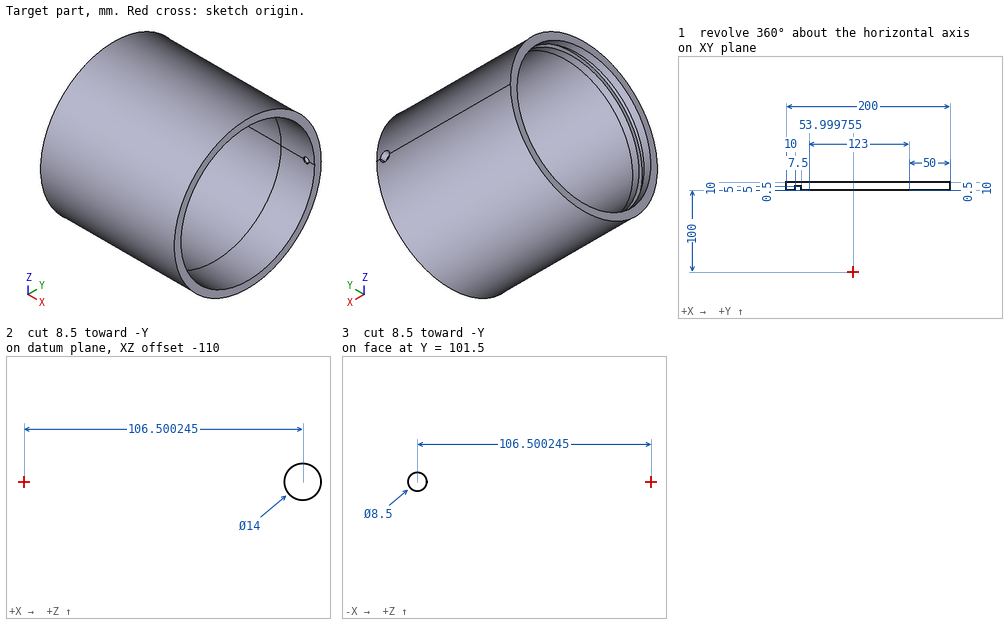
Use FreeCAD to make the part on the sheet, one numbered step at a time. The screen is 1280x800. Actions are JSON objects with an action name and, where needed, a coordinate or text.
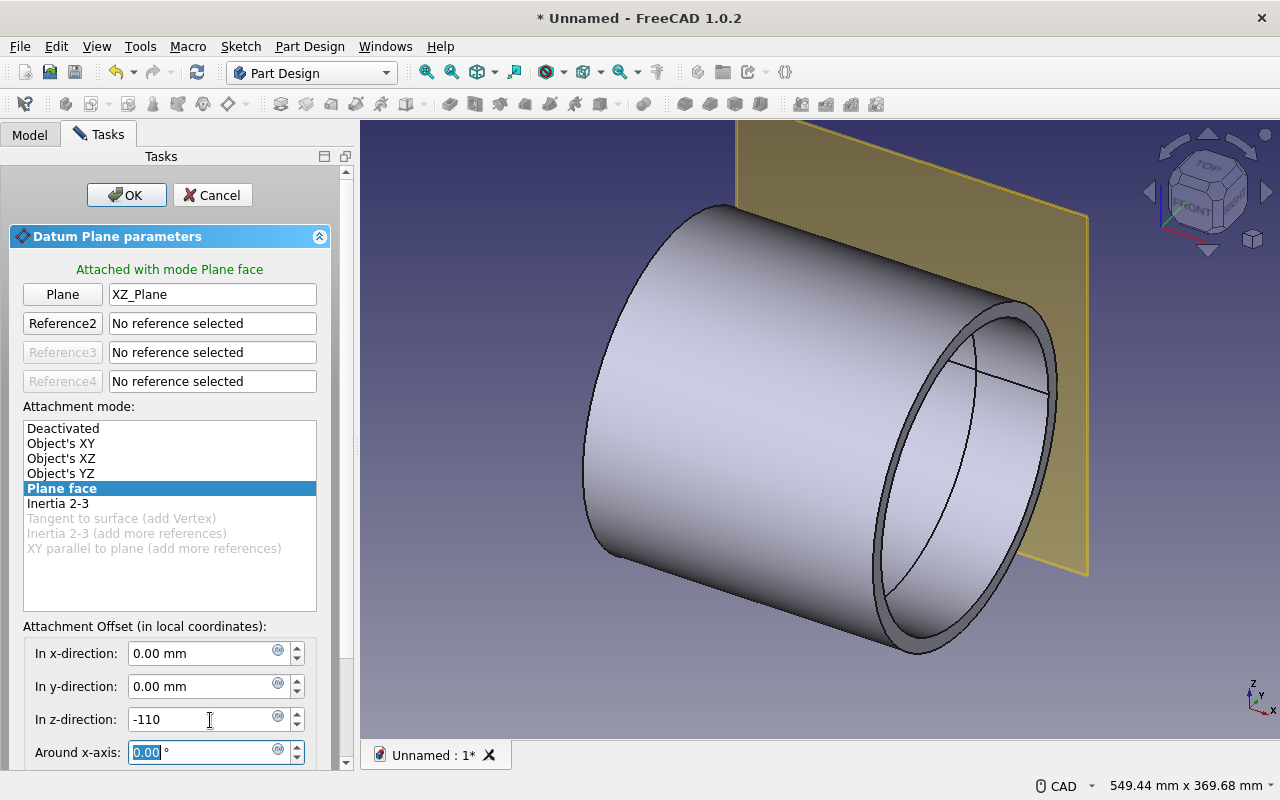
{"action": "left_click", "coordinate": [127, 195]}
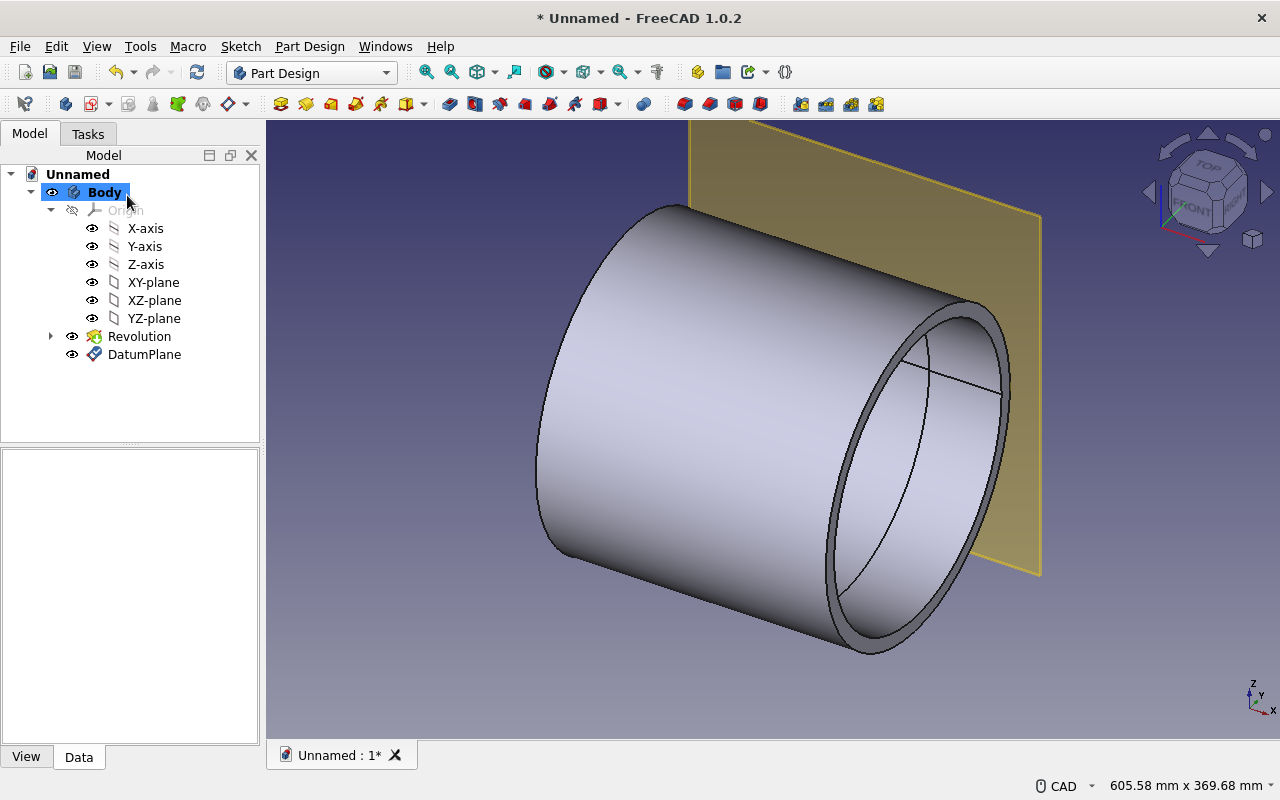
{"action": "left_click", "coordinate": [117, 354]}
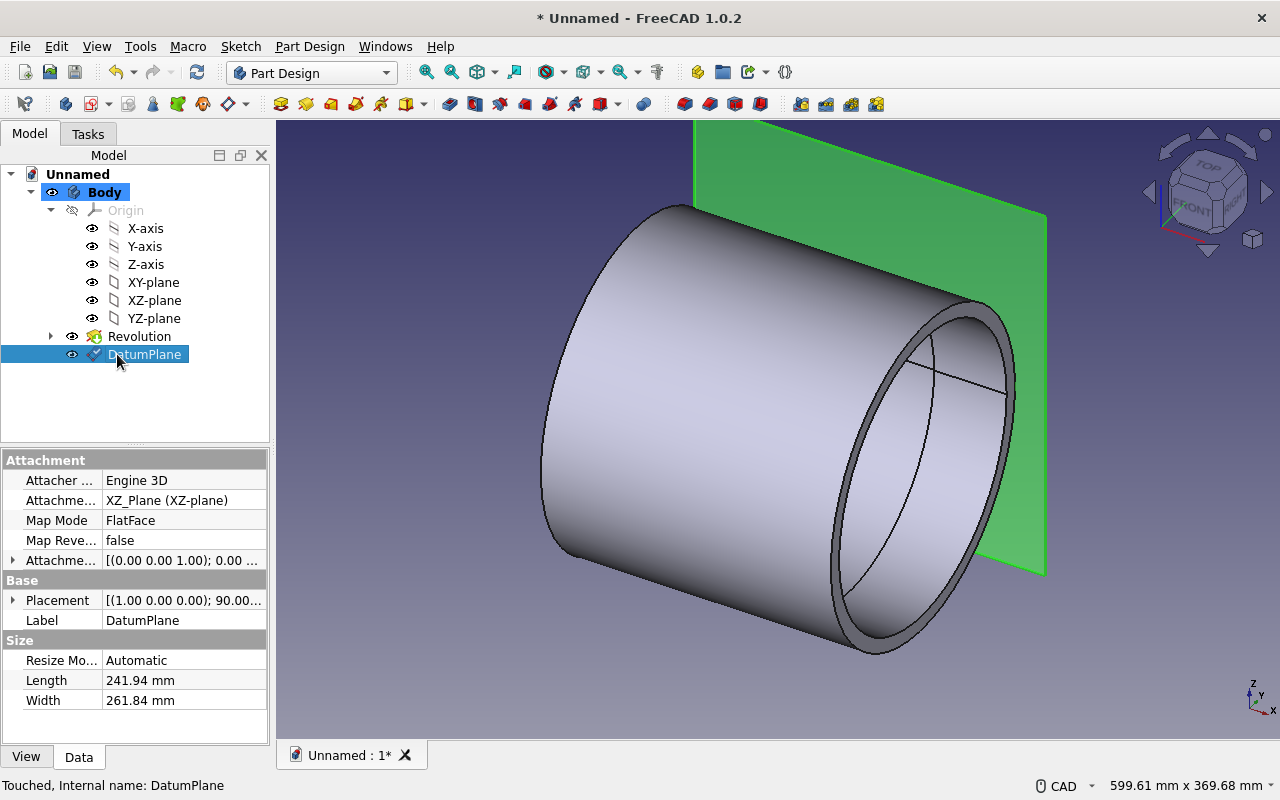
{"action": "left_click", "coordinate": [90, 104]}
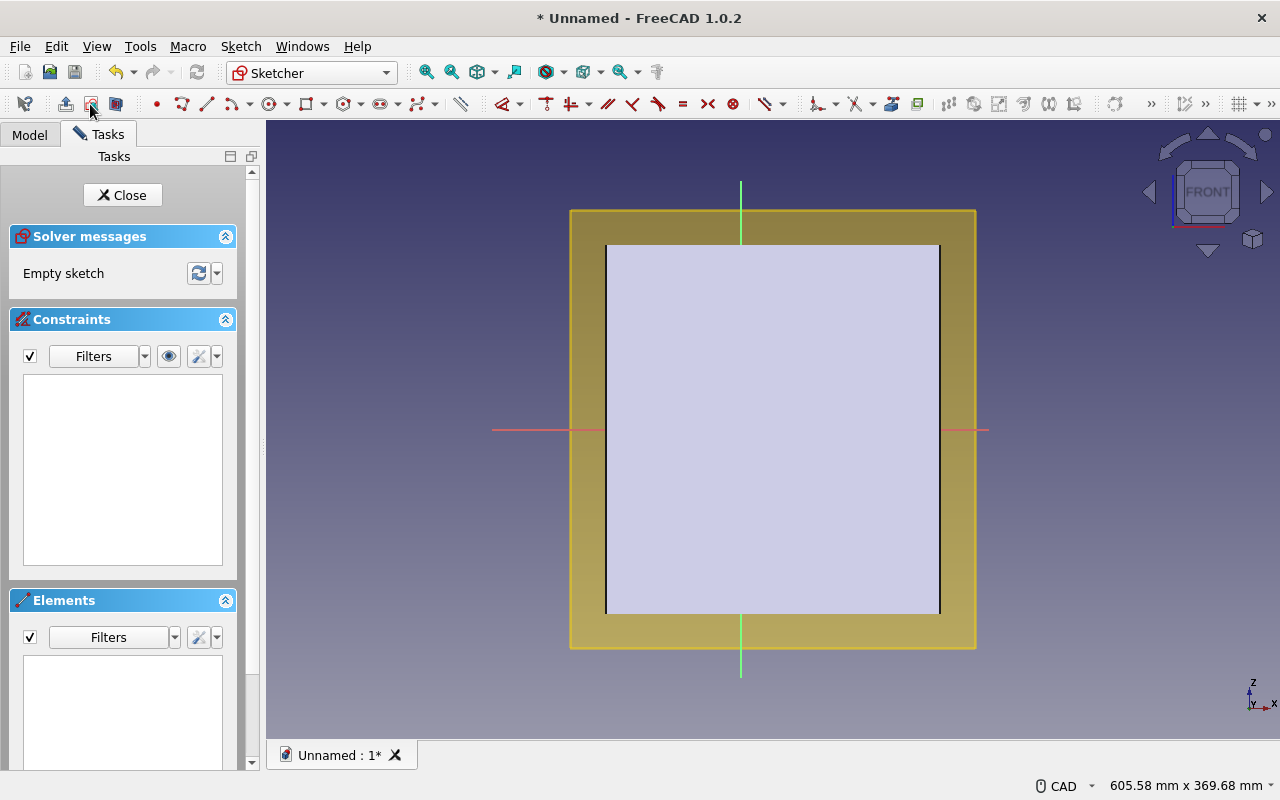
{"action": "left_click", "coordinate": [116, 104]}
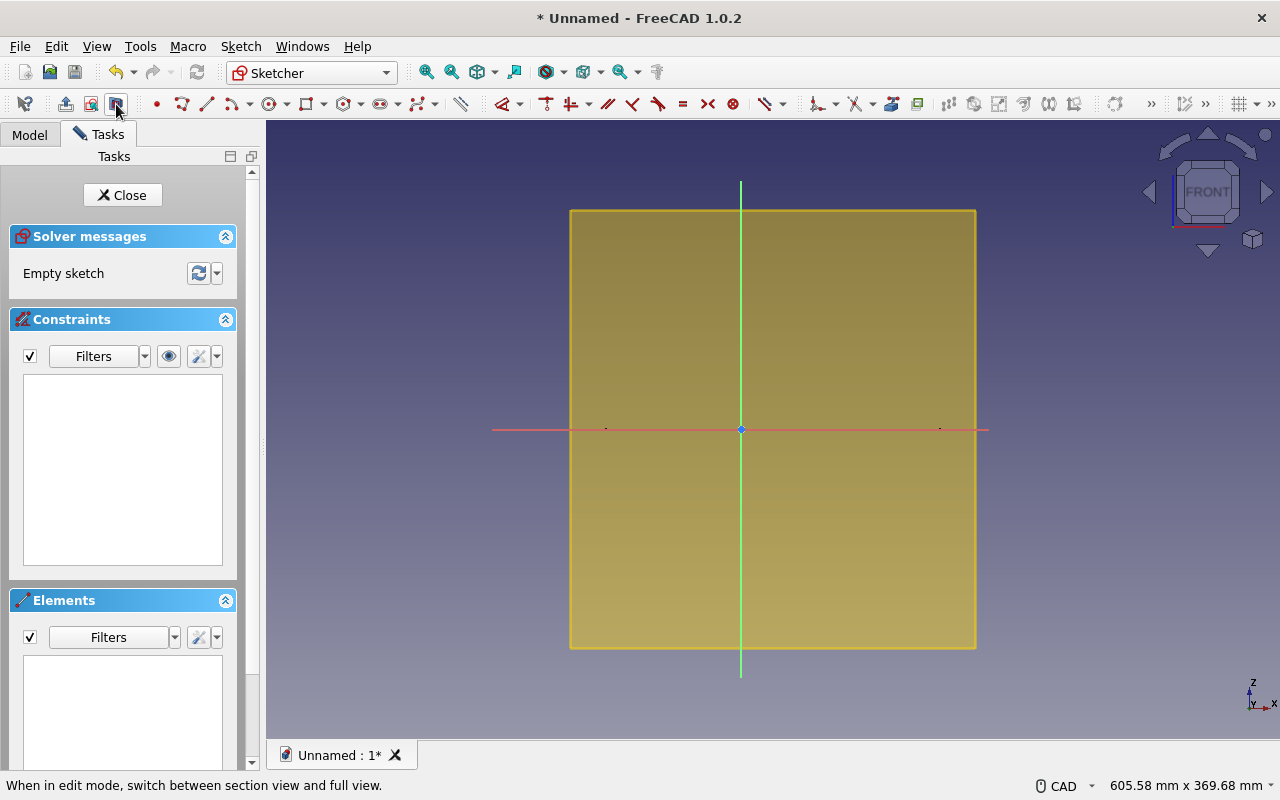
{"action": "scroll", "coordinate": [933, 430], "scroll_direction": "up", "scroll_amount": 14}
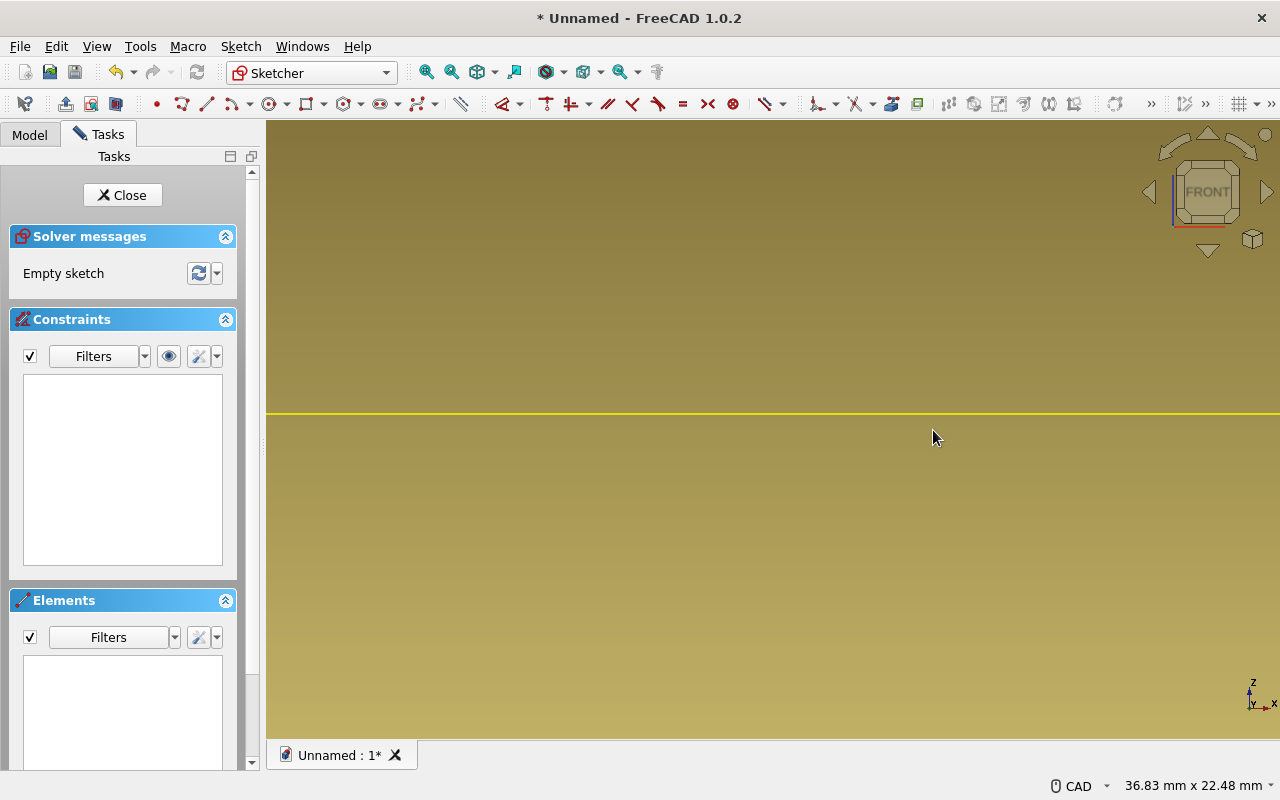
{"action": "left_click", "coordinate": [268, 104]}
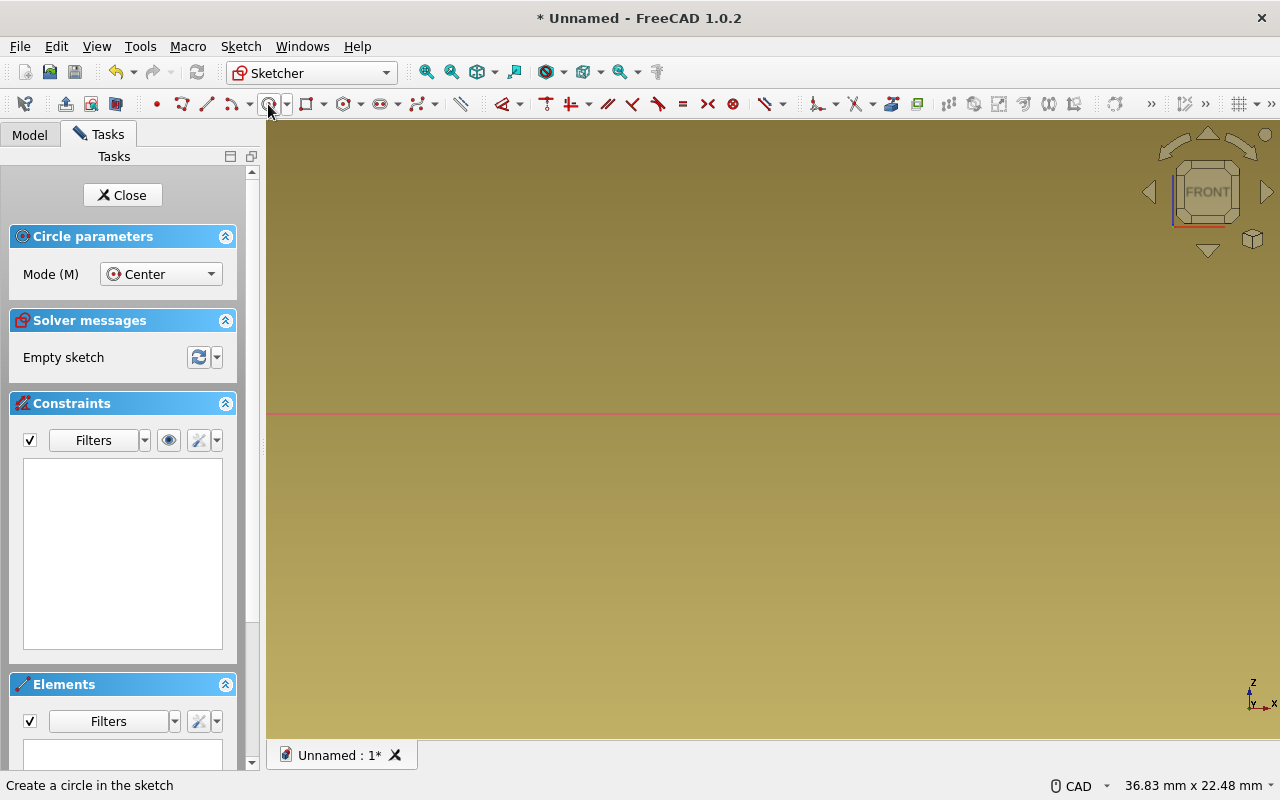
{"action": "left_click", "coordinate": [701, 414]}
{"action": "mouse_move", "coordinate": [837, 278]}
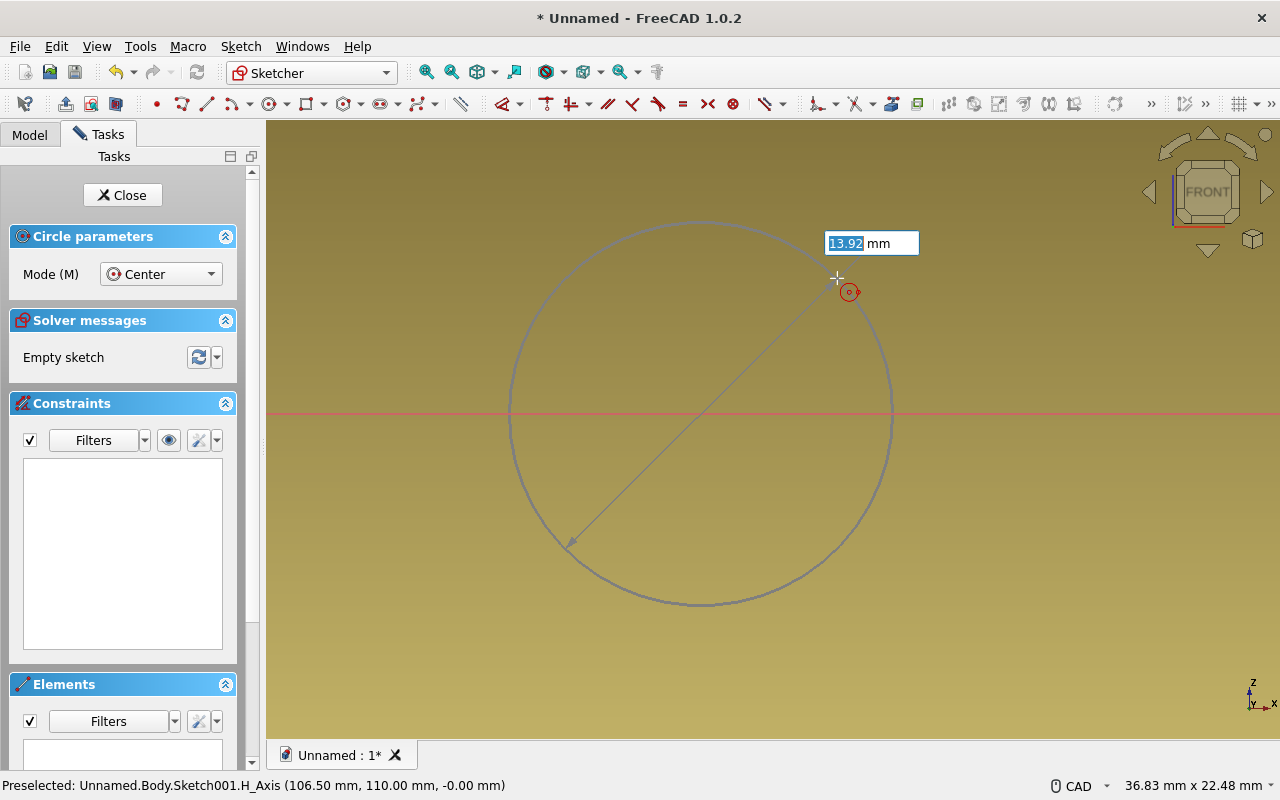
{"action": "type", "text": "14"}
{"action": "key", "text": "Return"}
{"action": "key", "text": "Escape"}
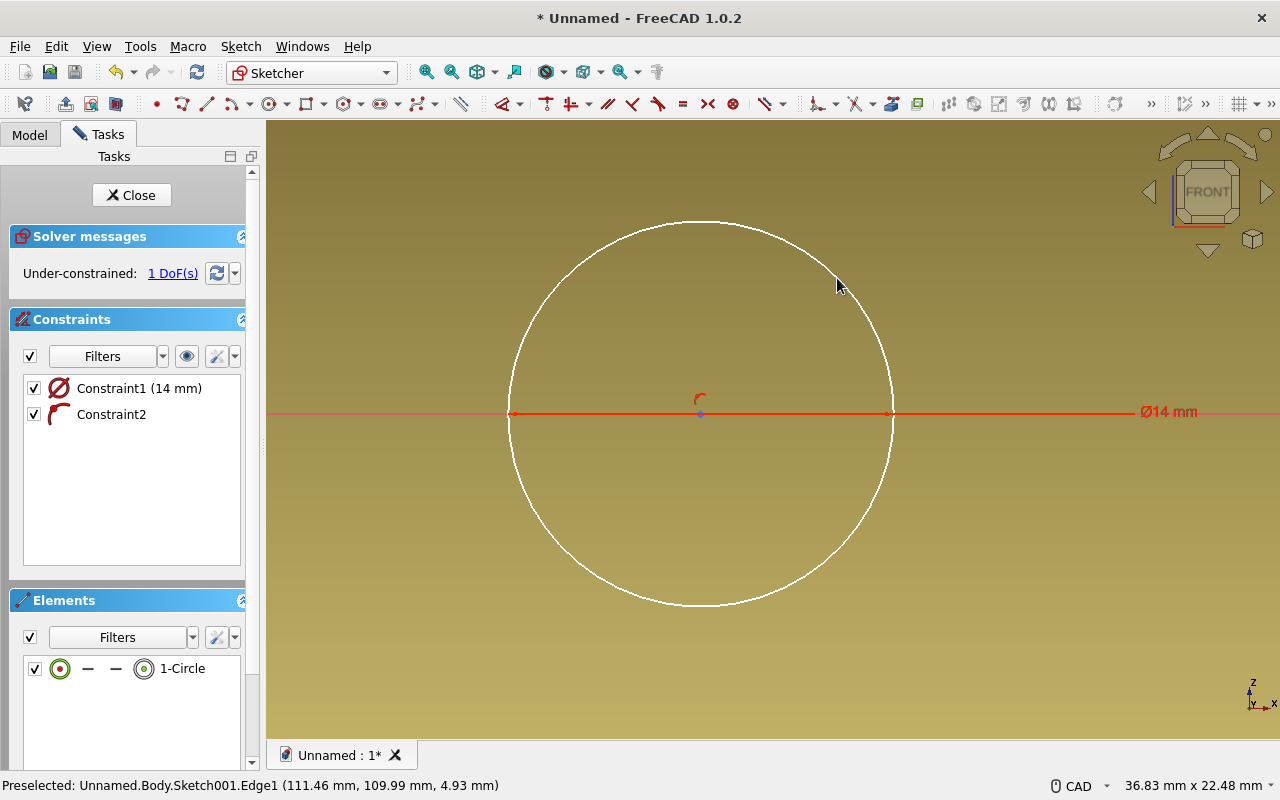
{"action": "key", "text": "d"}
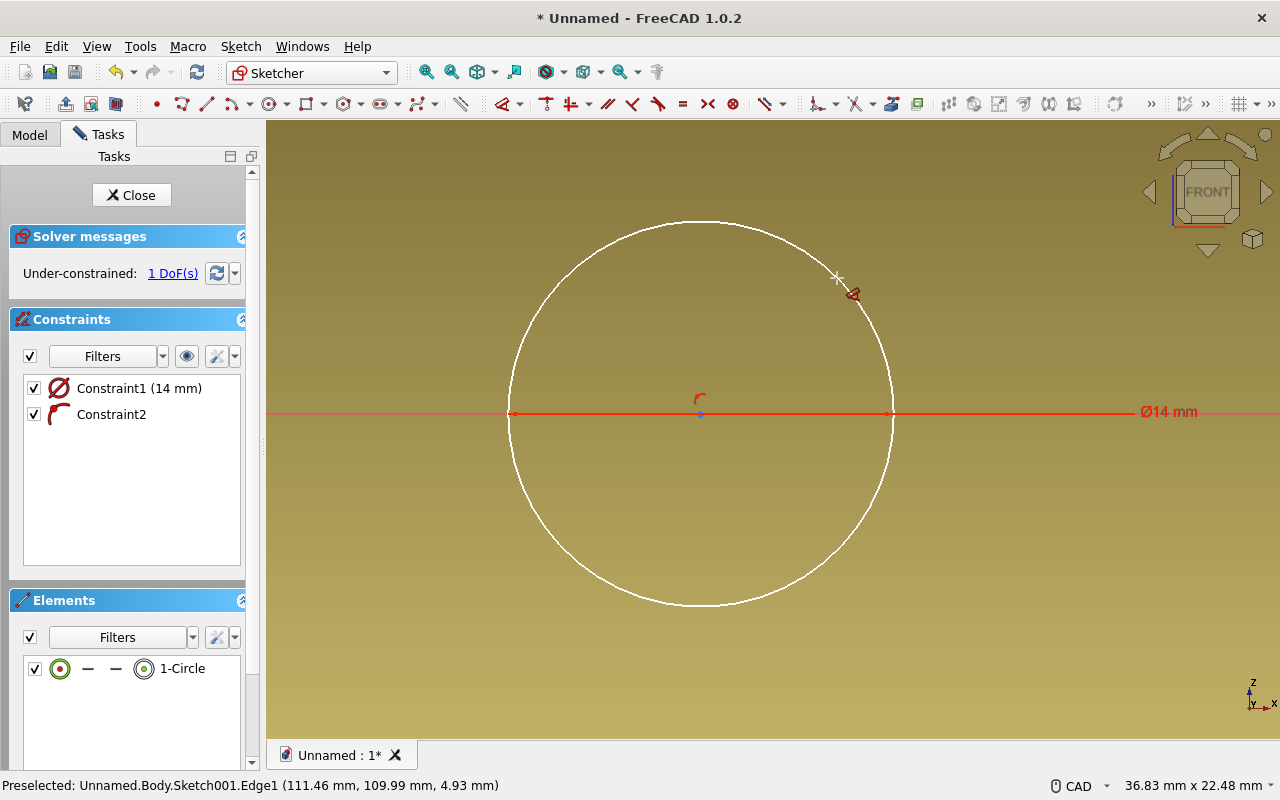
{"action": "left_click", "coordinate": [701, 414]}
{"action": "left_click", "coordinate": [497, 448]}